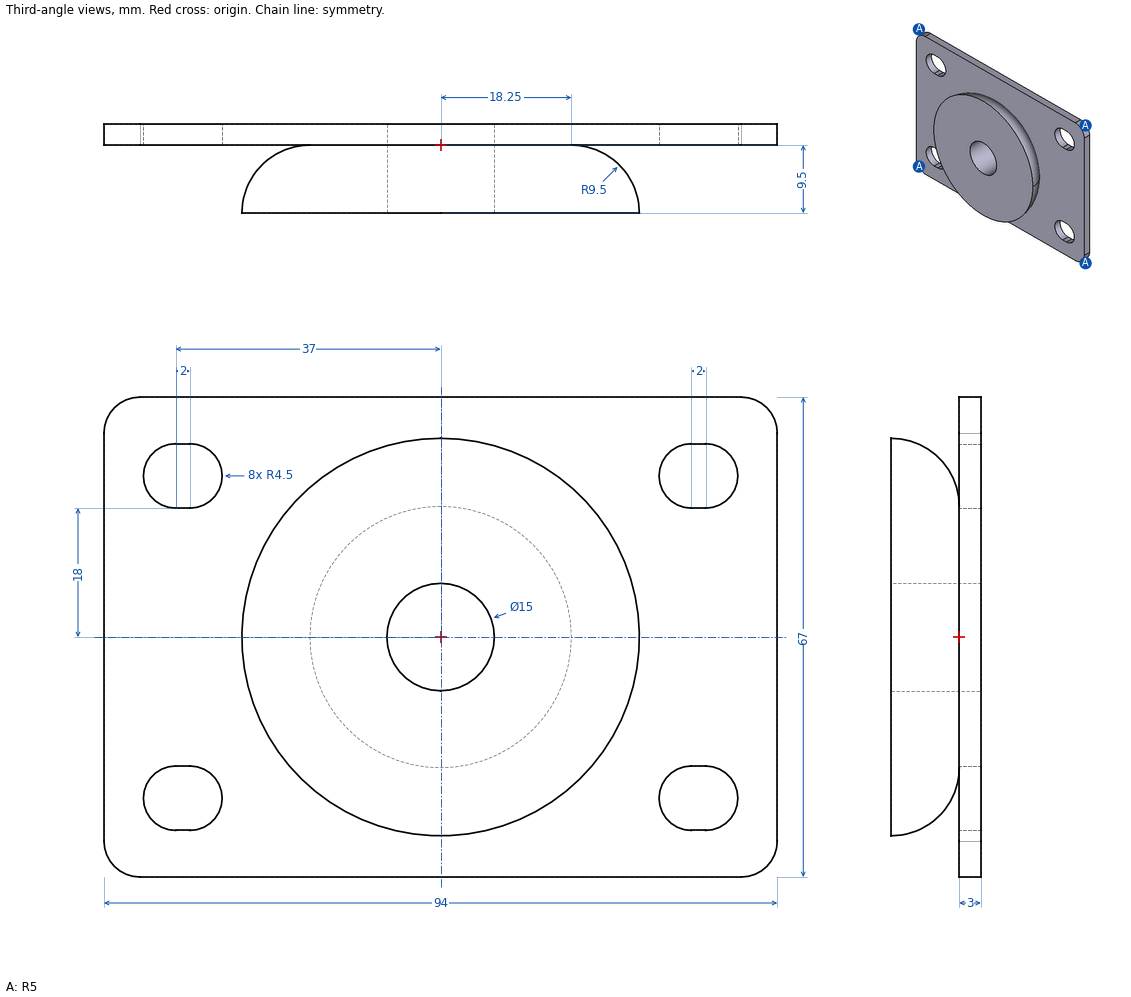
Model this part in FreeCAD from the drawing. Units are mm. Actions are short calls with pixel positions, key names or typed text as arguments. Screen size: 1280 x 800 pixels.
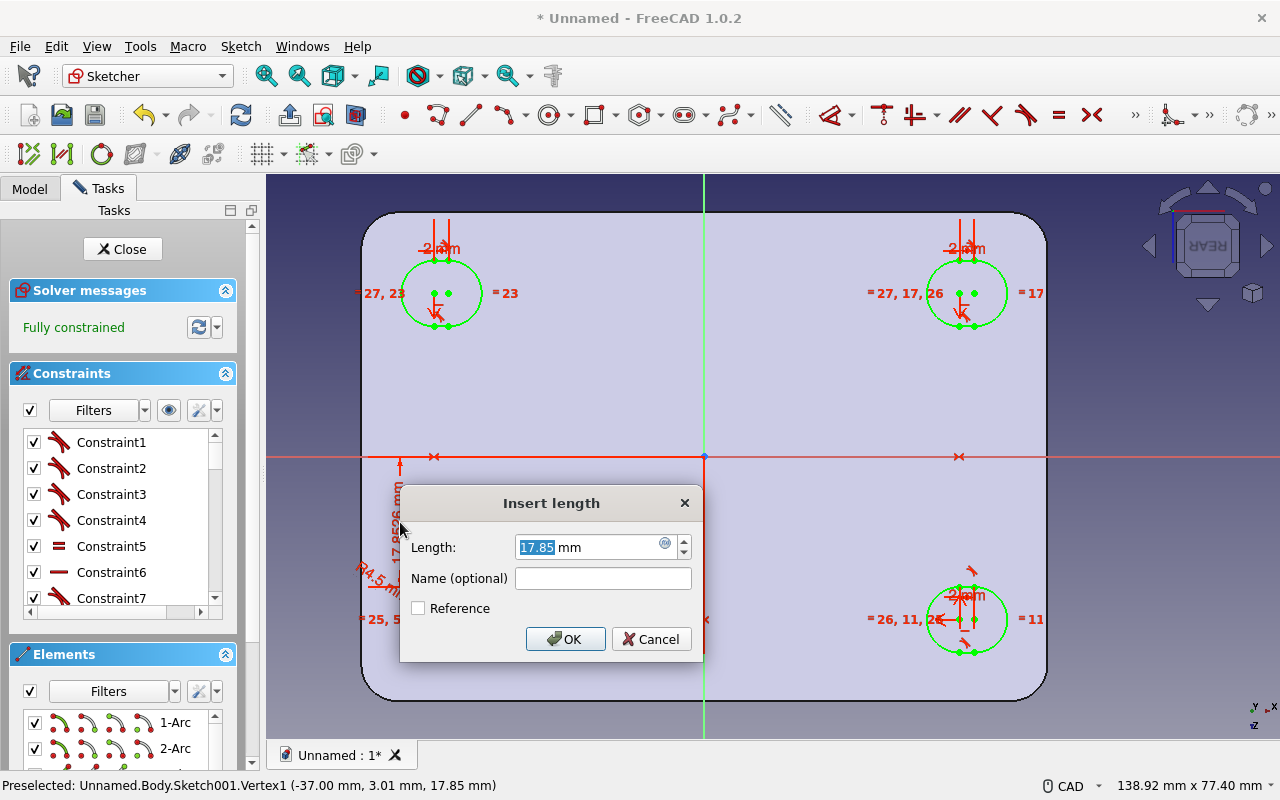
text(18)
key(Return)
key(Escape)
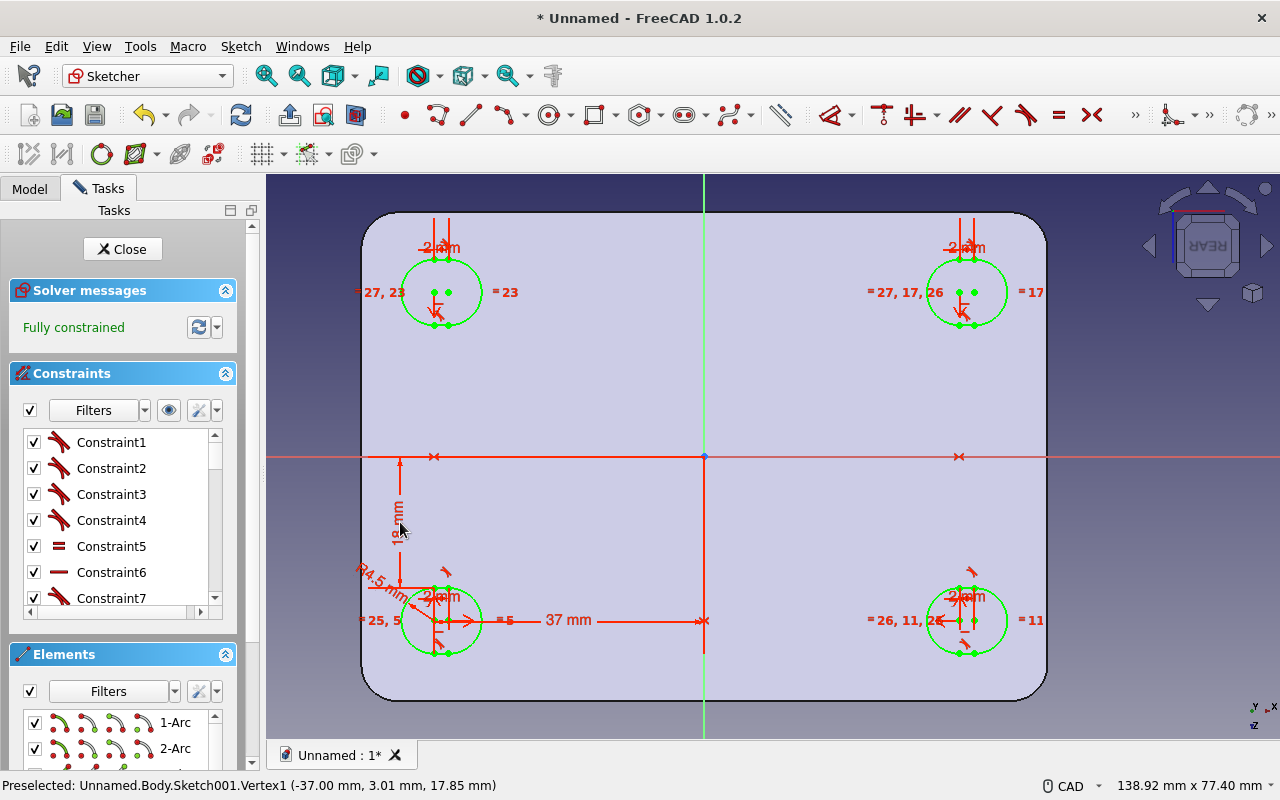
click(123, 249)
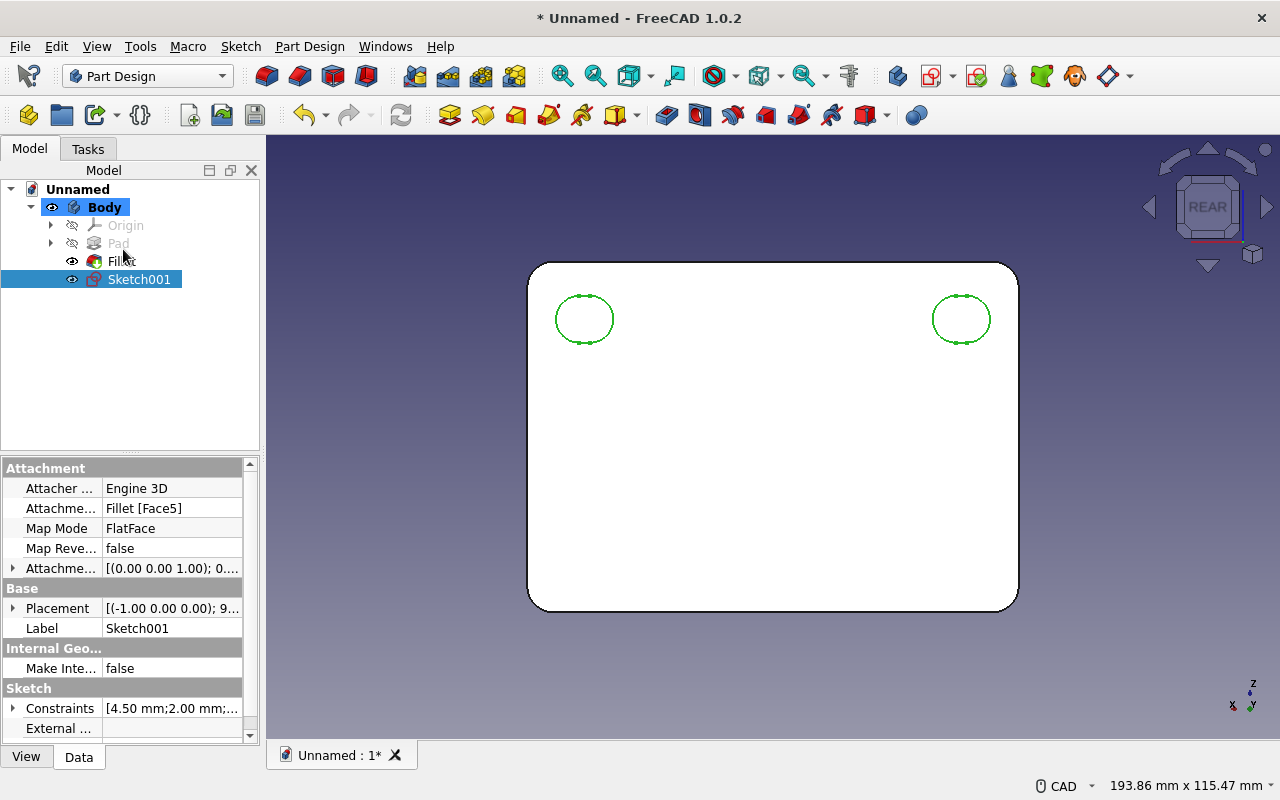
click(667, 116)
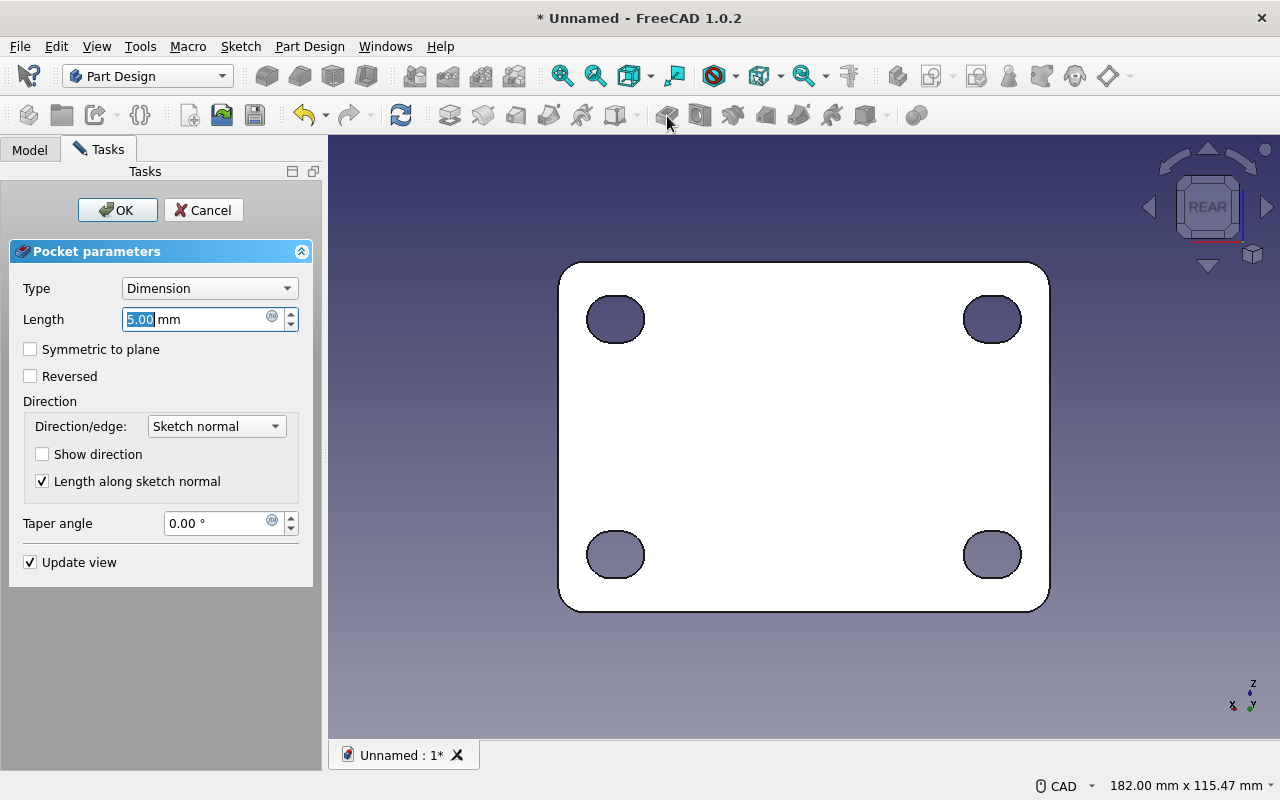
click(210, 288)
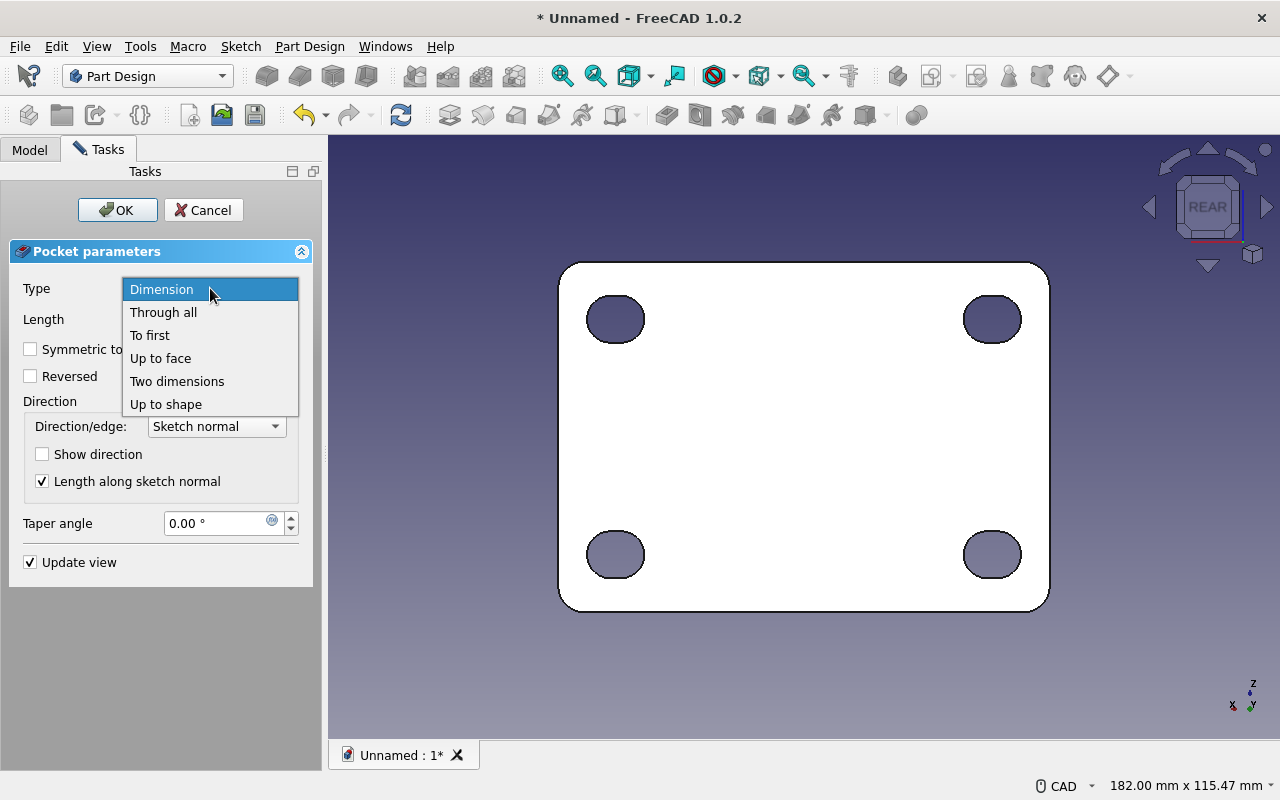
click(208, 312)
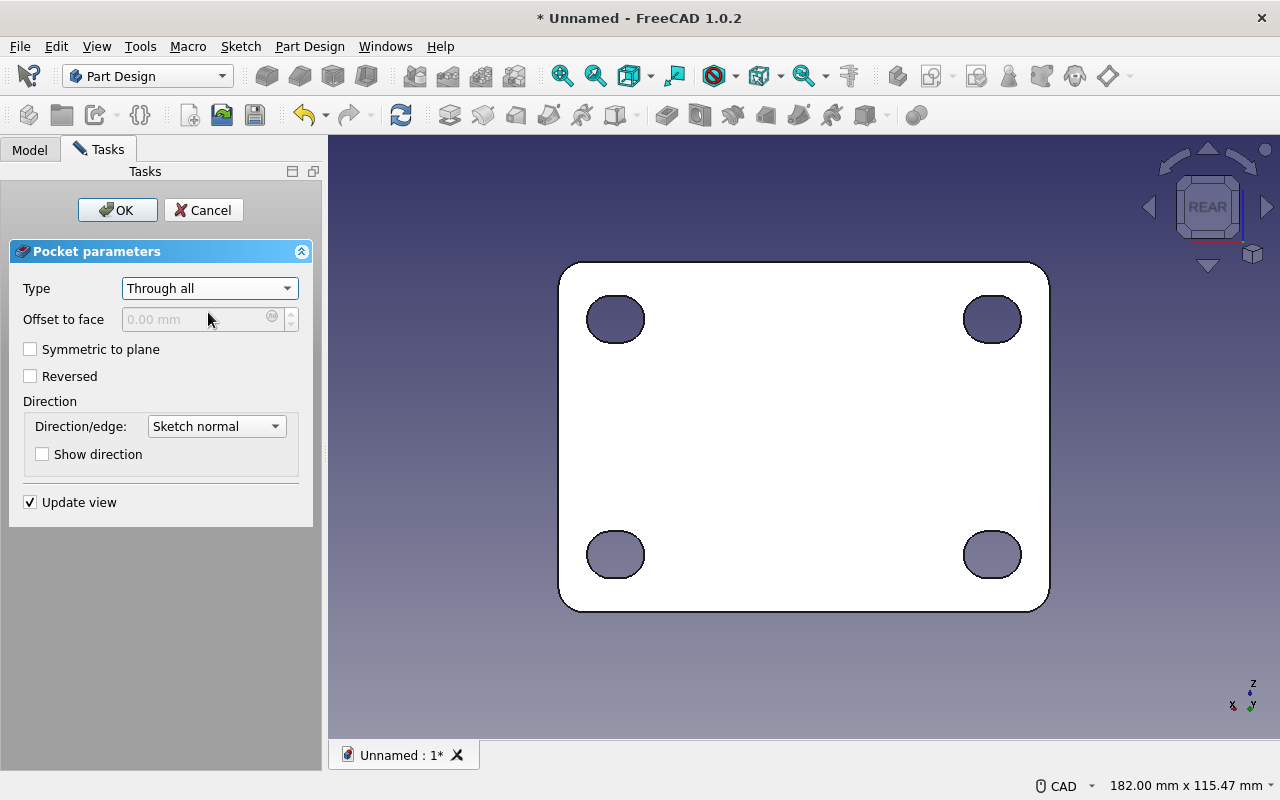
click(118, 210)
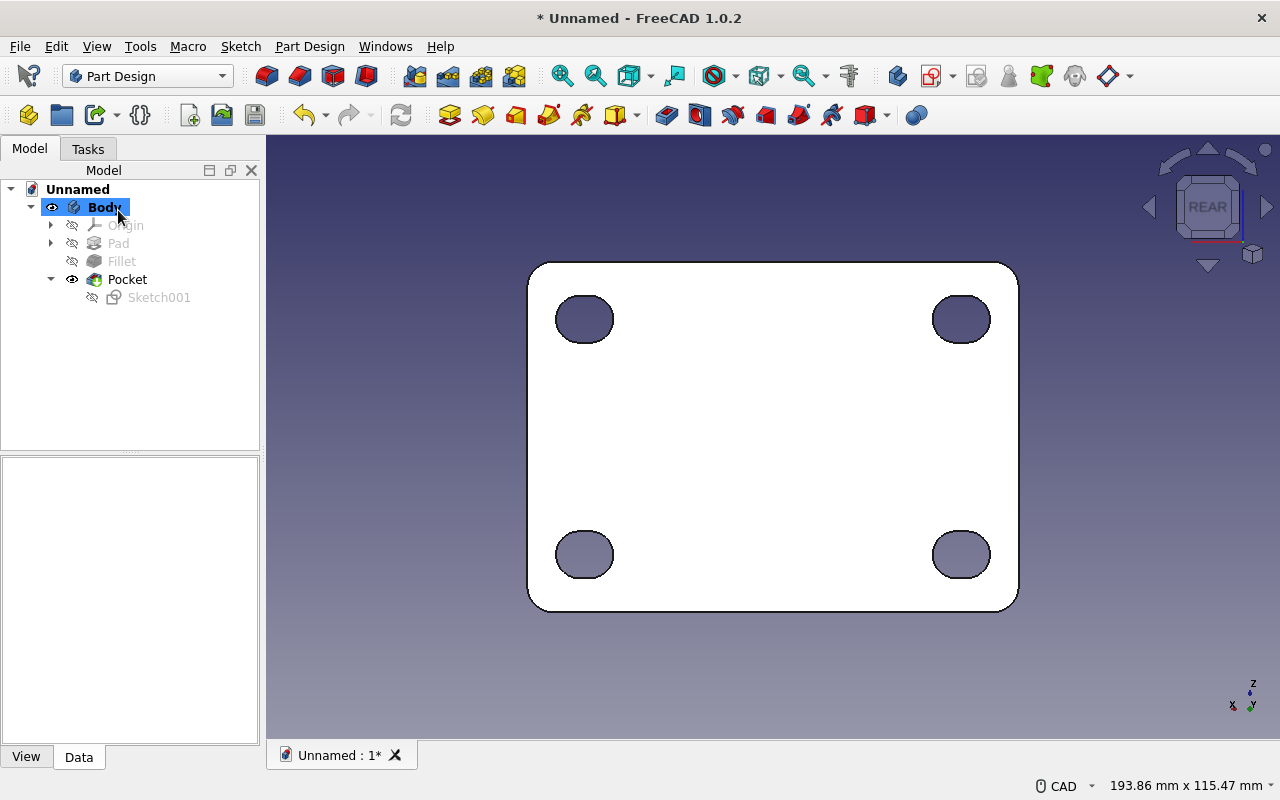
click(930, 76)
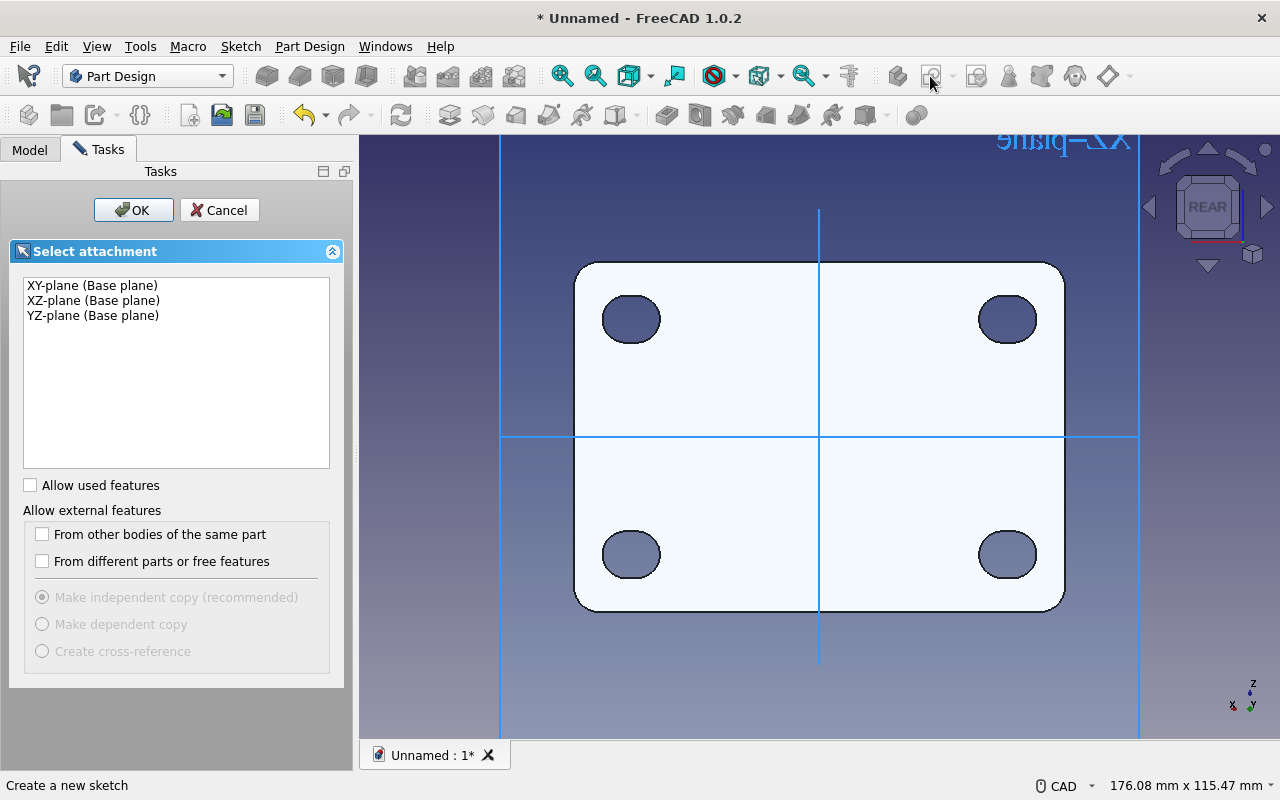
click(84, 286)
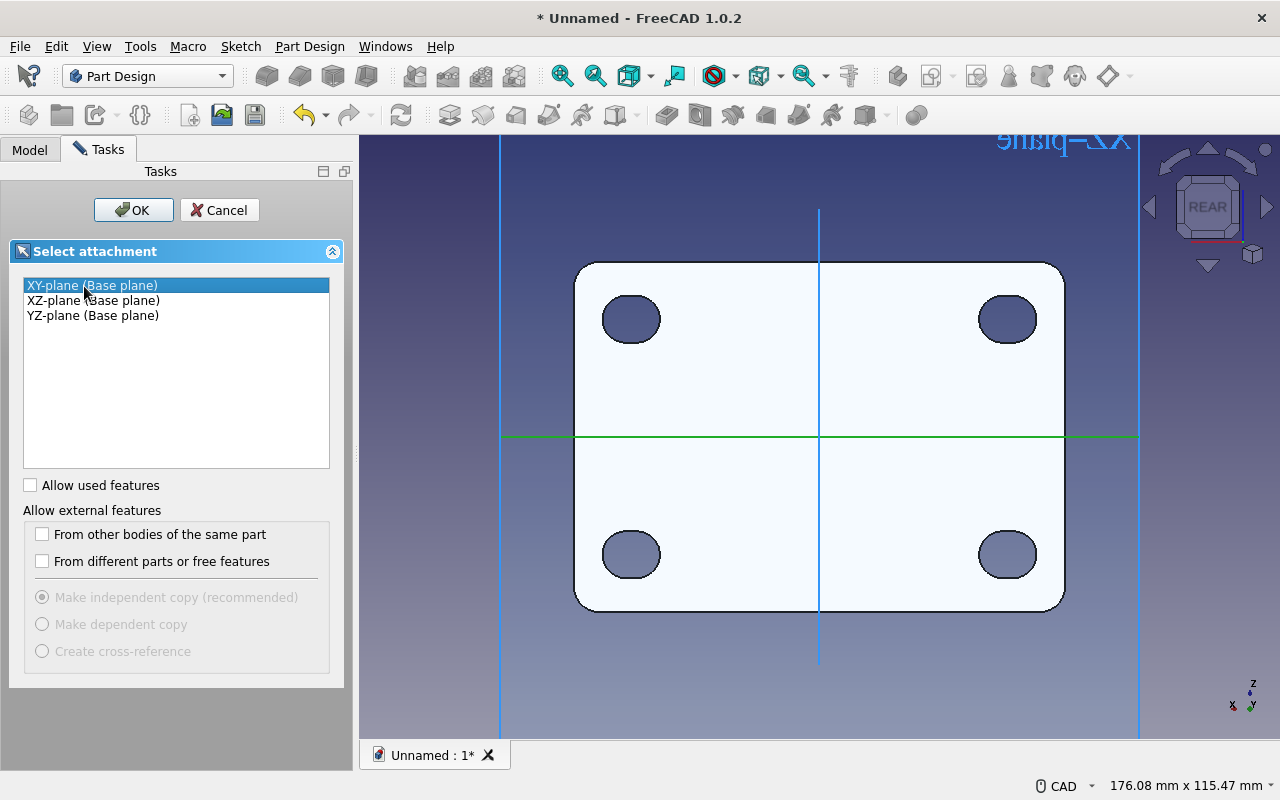
click(134, 210)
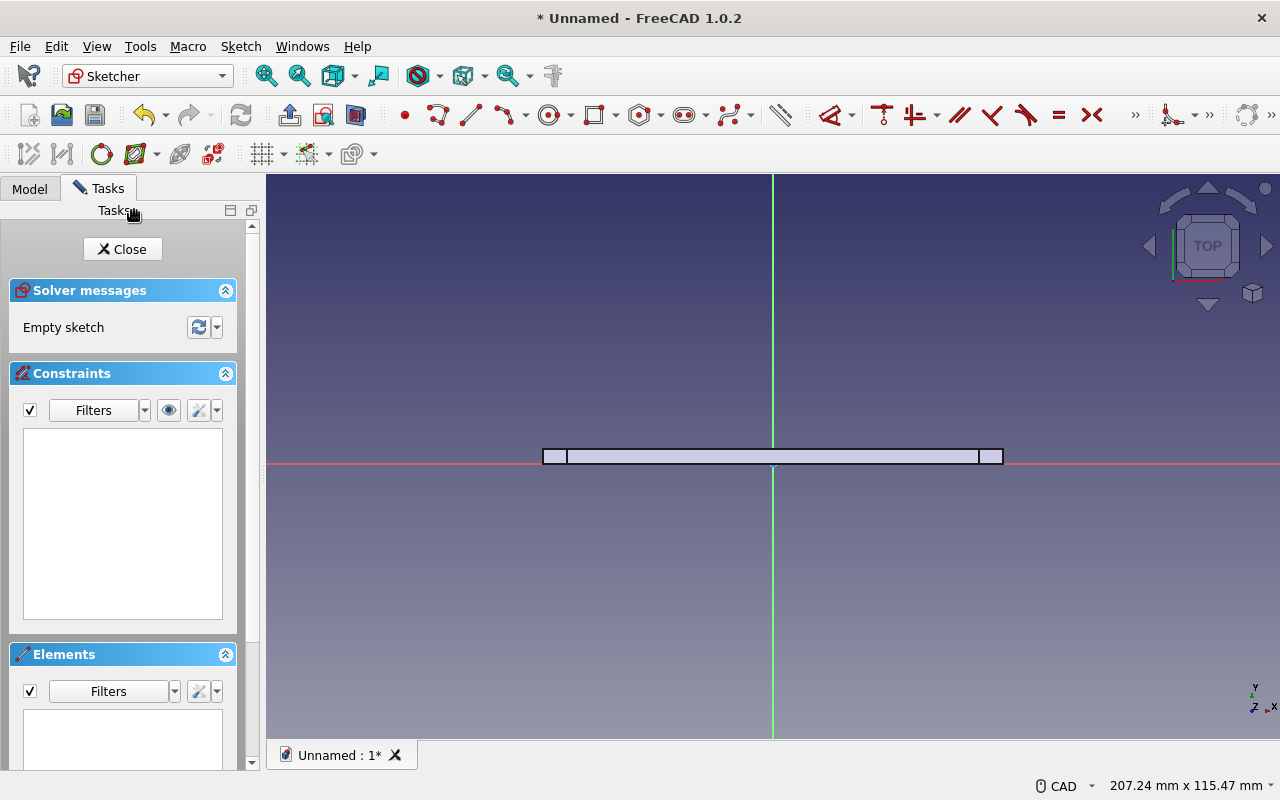
key(q)
key(s)